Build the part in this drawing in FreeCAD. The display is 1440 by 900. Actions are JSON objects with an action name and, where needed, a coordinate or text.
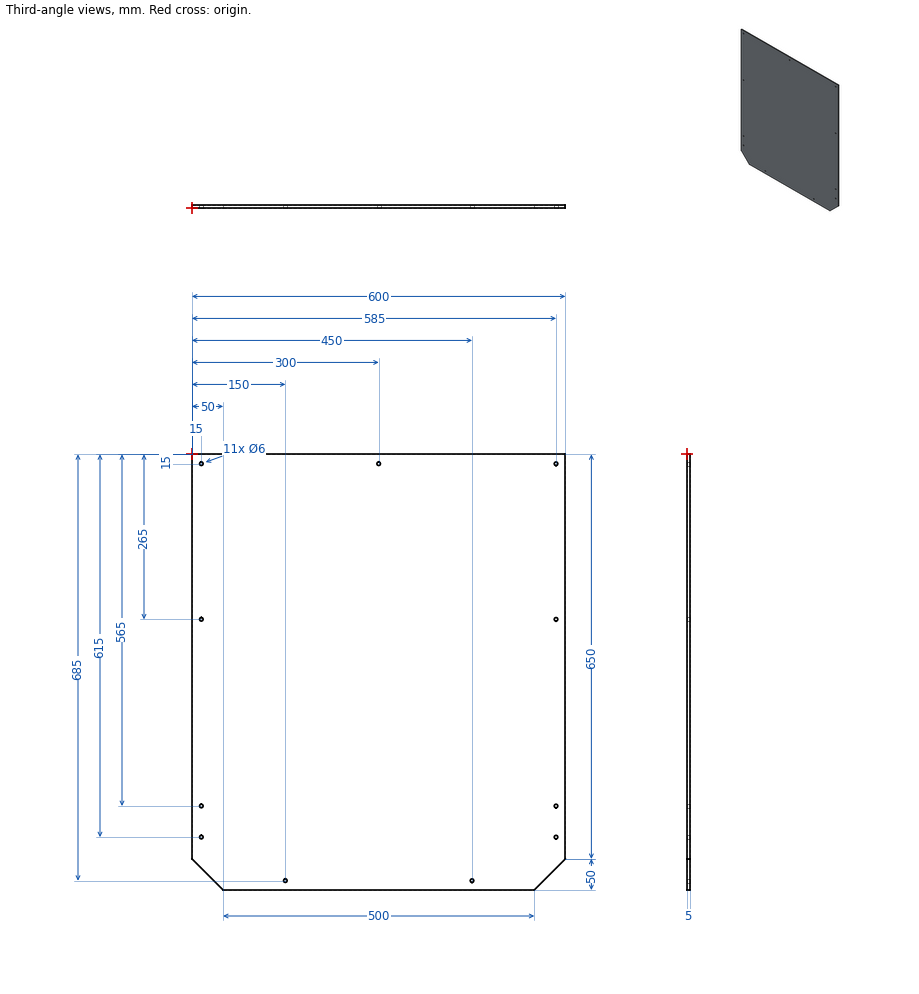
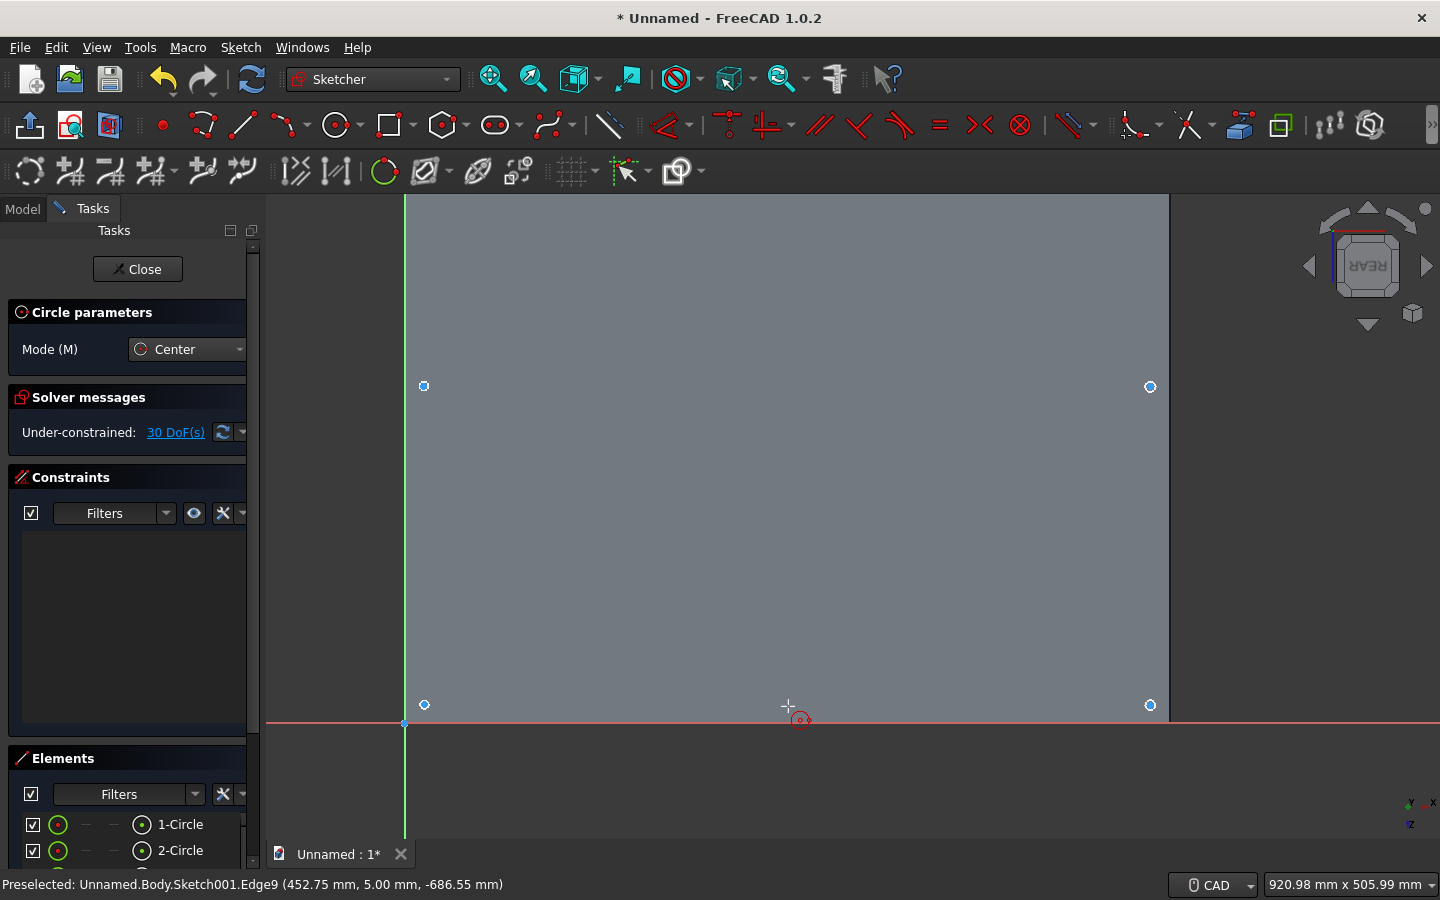
{"action": "left_click", "coordinate": [787, 704]}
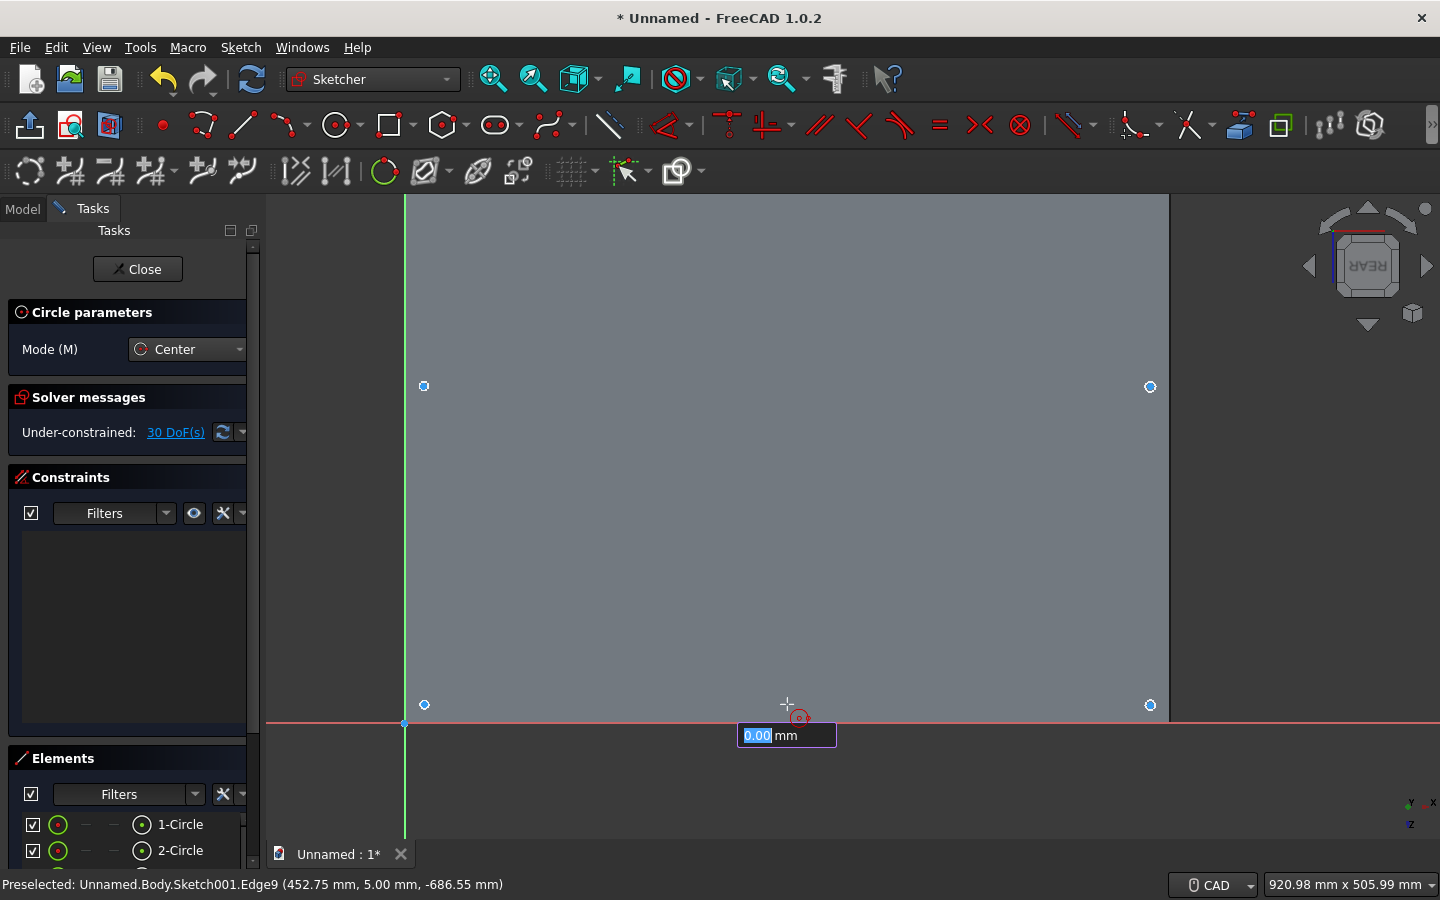
{"action": "scroll", "coordinate": [790, 701], "scroll_direction": "up", "scroll_amount": 8}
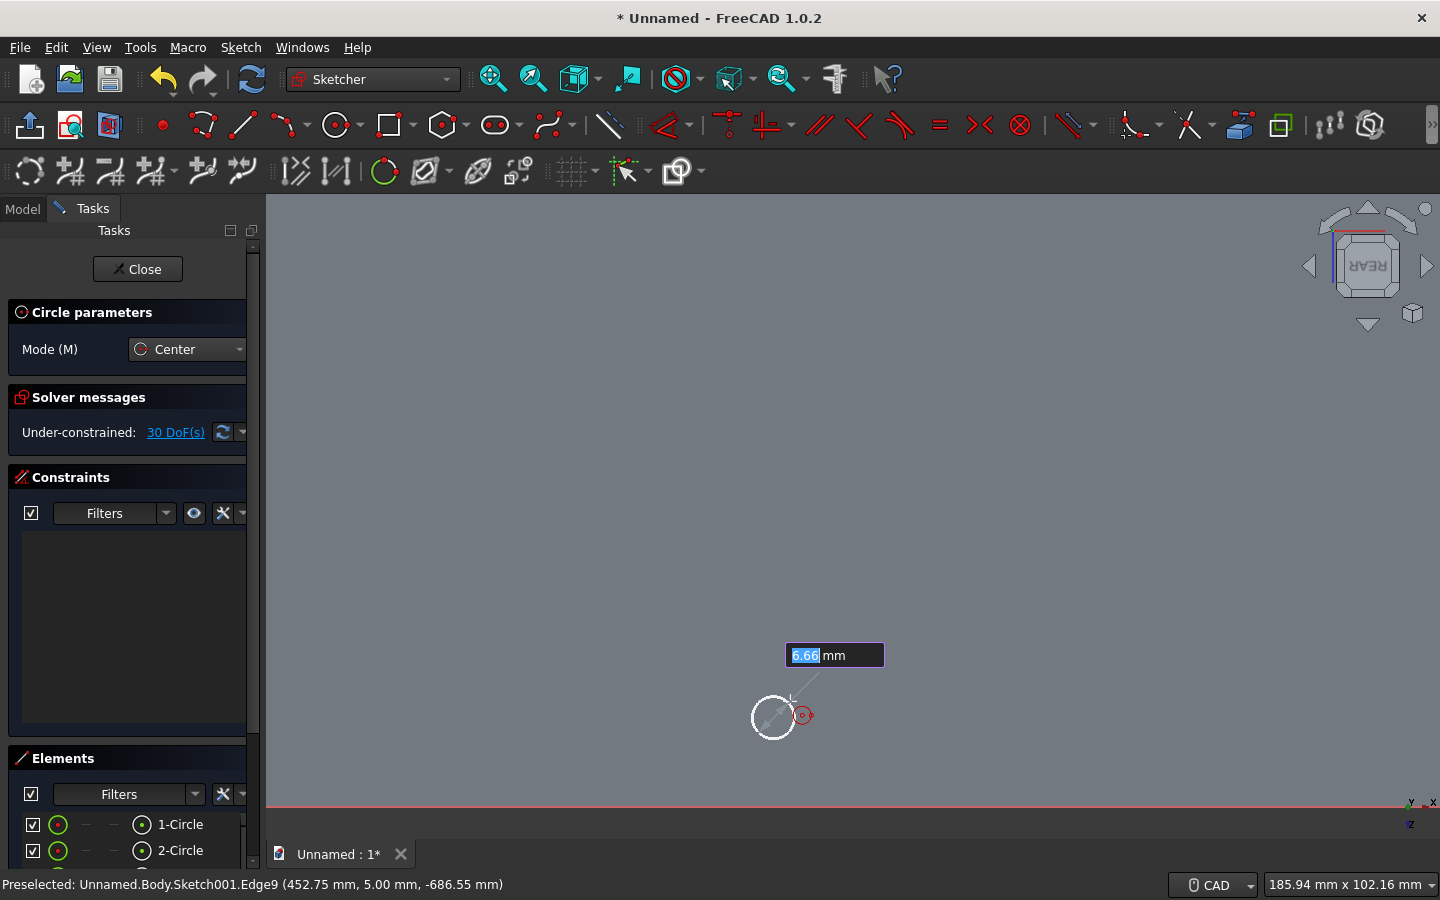
{"action": "left_click", "coordinate": [789, 699]}
{"action": "key", "text": "Escape"}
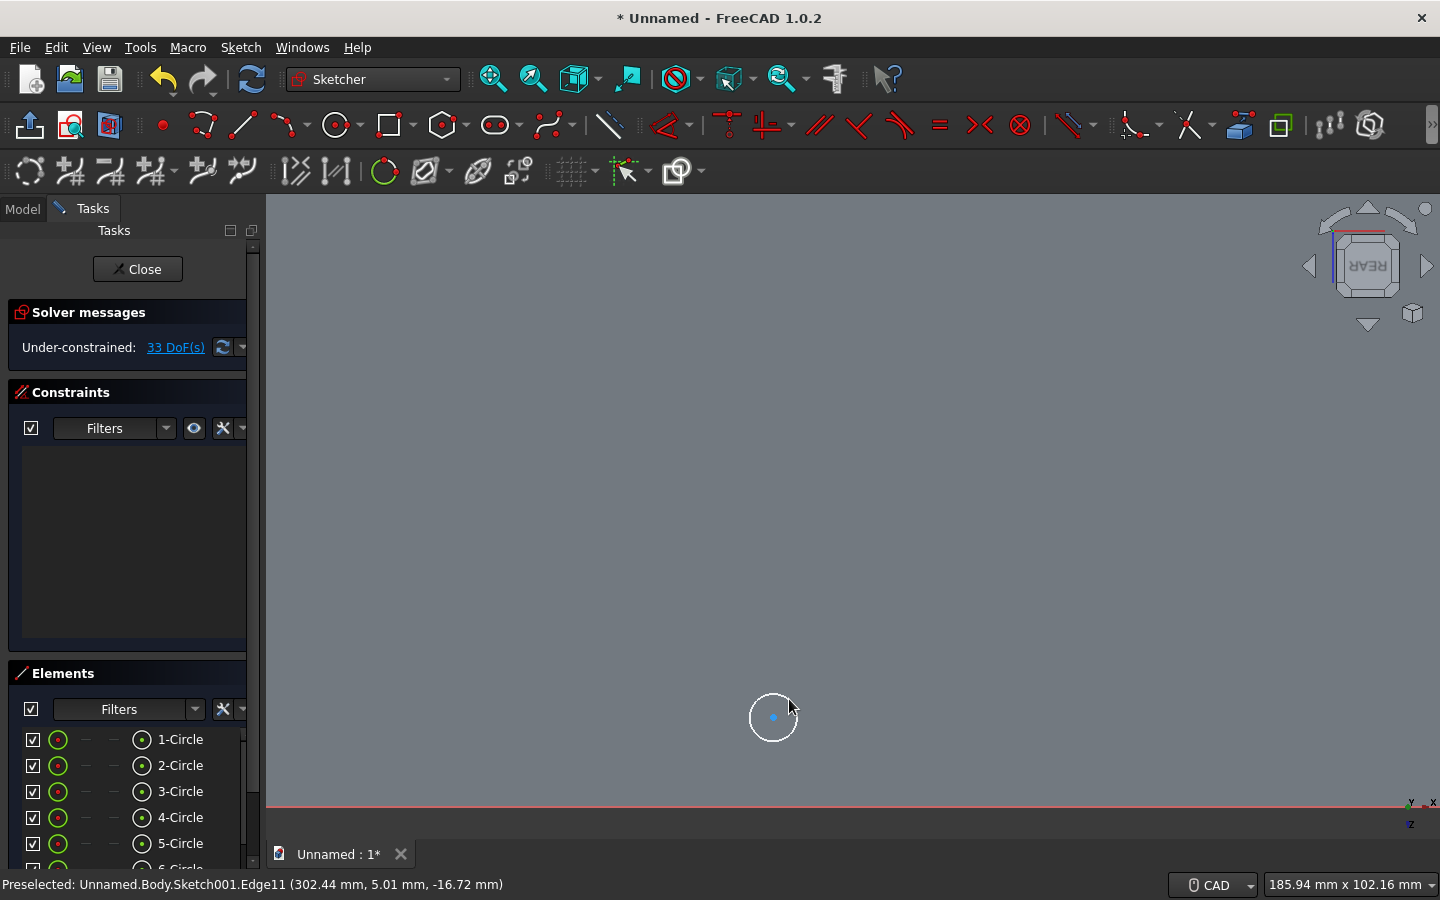
{"action": "scroll", "coordinate": [789, 704], "scroll_direction": "down", "scroll_amount": 12}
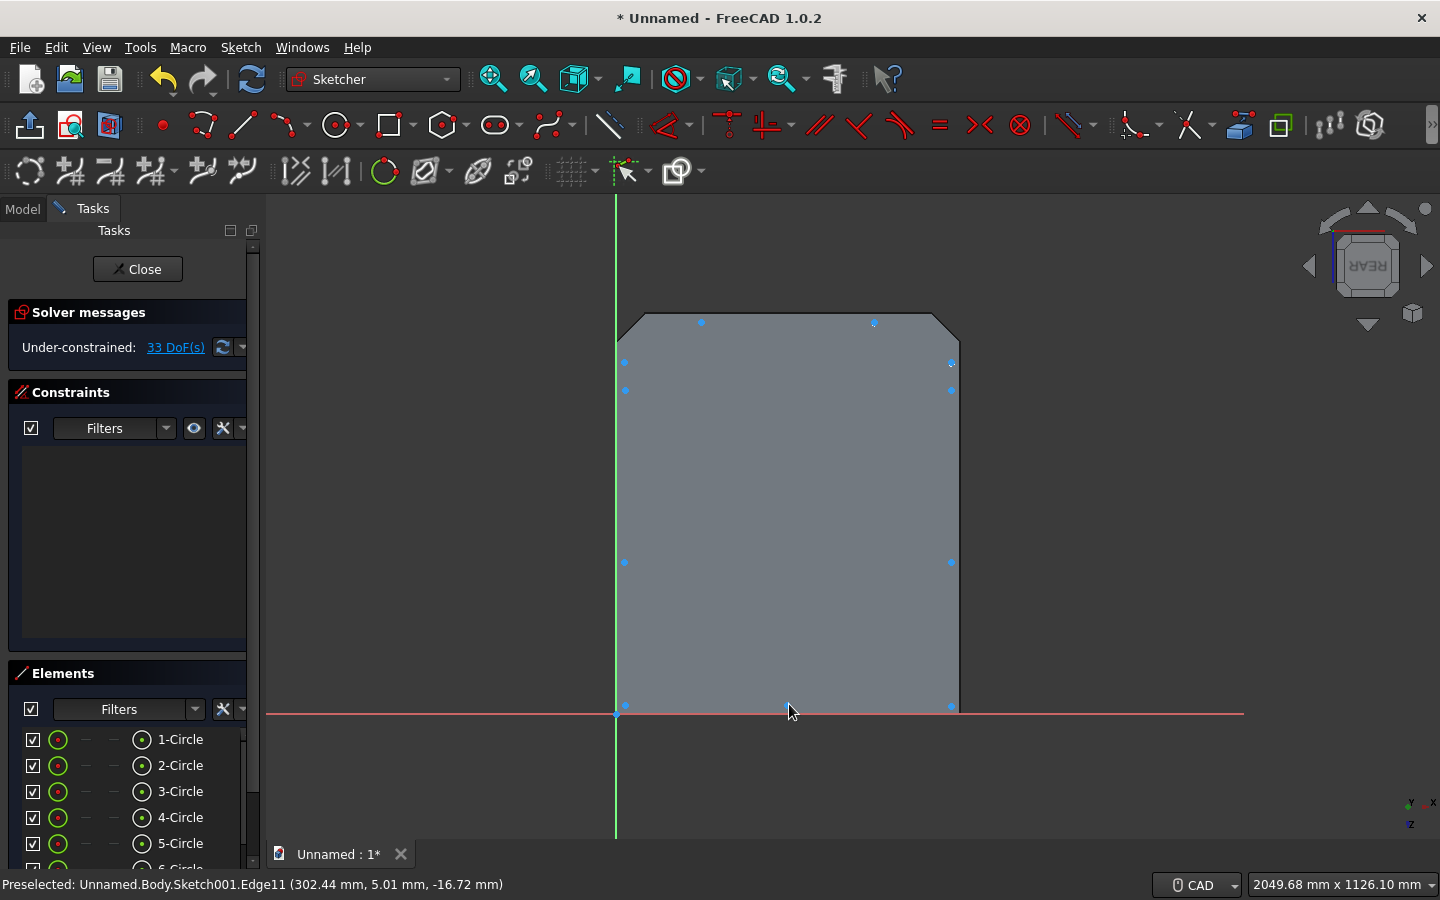
{"action": "scroll", "coordinate": [626, 705], "scroll_direction": "up", "scroll_amount": 10}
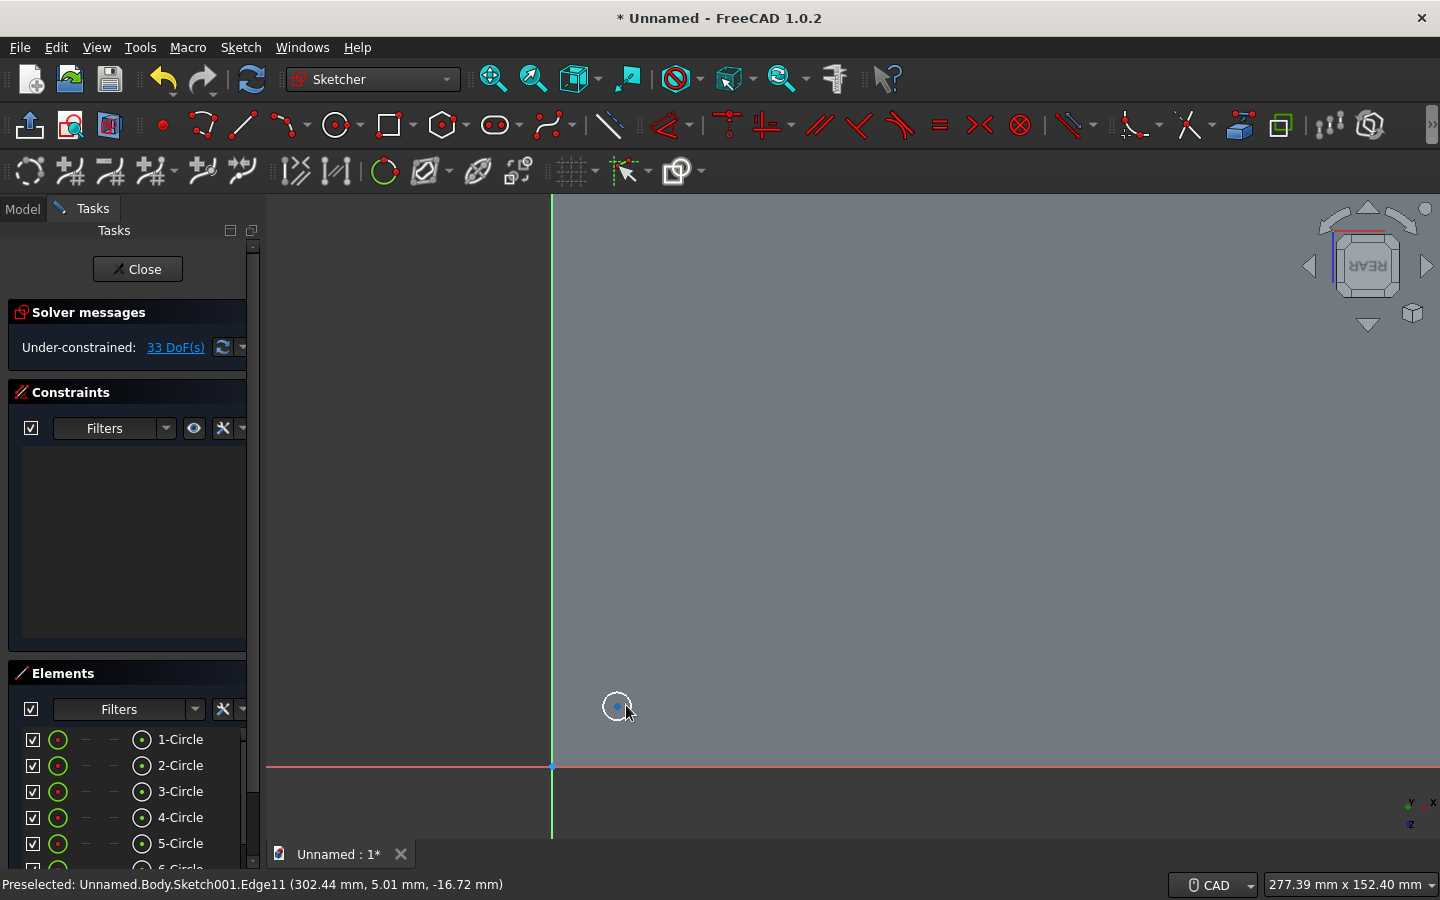
{"action": "left_click", "coordinate": [627, 696]}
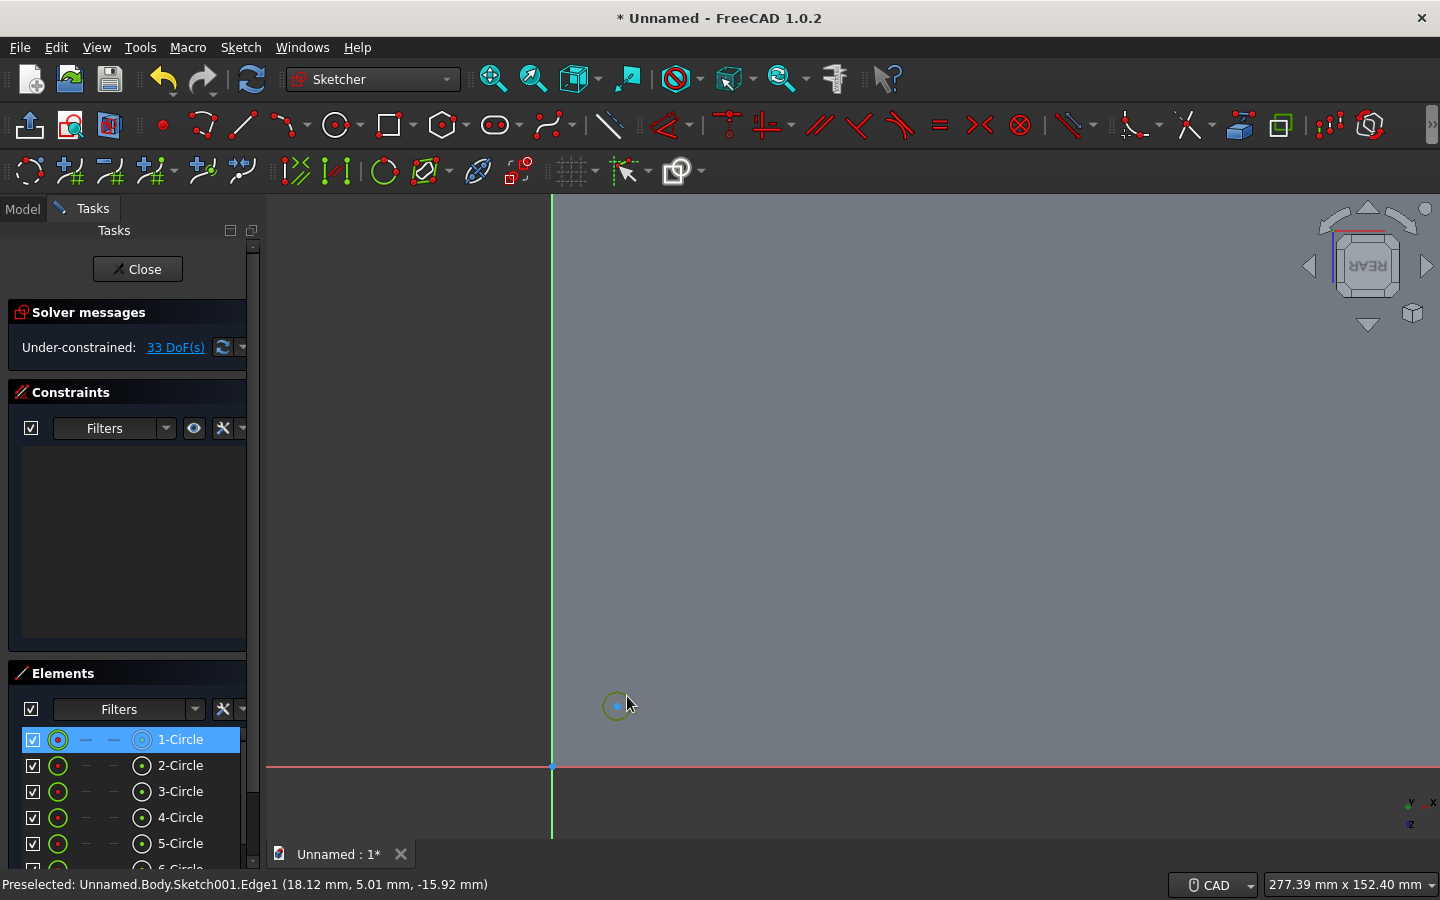
{"action": "scroll", "coordinate": [626, 705], "scroll_direction": "down", "scroll_amount": 10}